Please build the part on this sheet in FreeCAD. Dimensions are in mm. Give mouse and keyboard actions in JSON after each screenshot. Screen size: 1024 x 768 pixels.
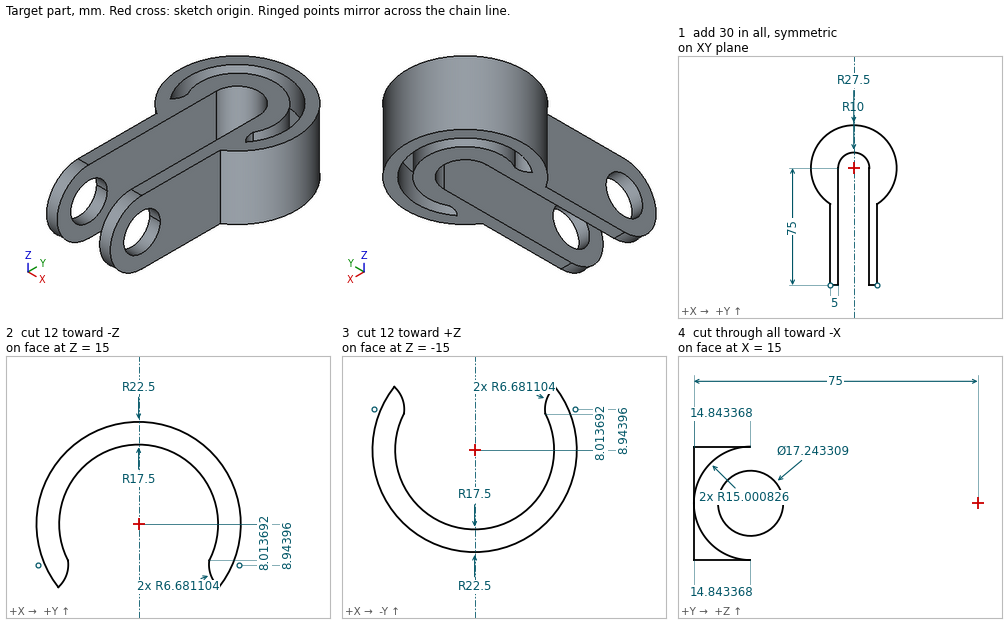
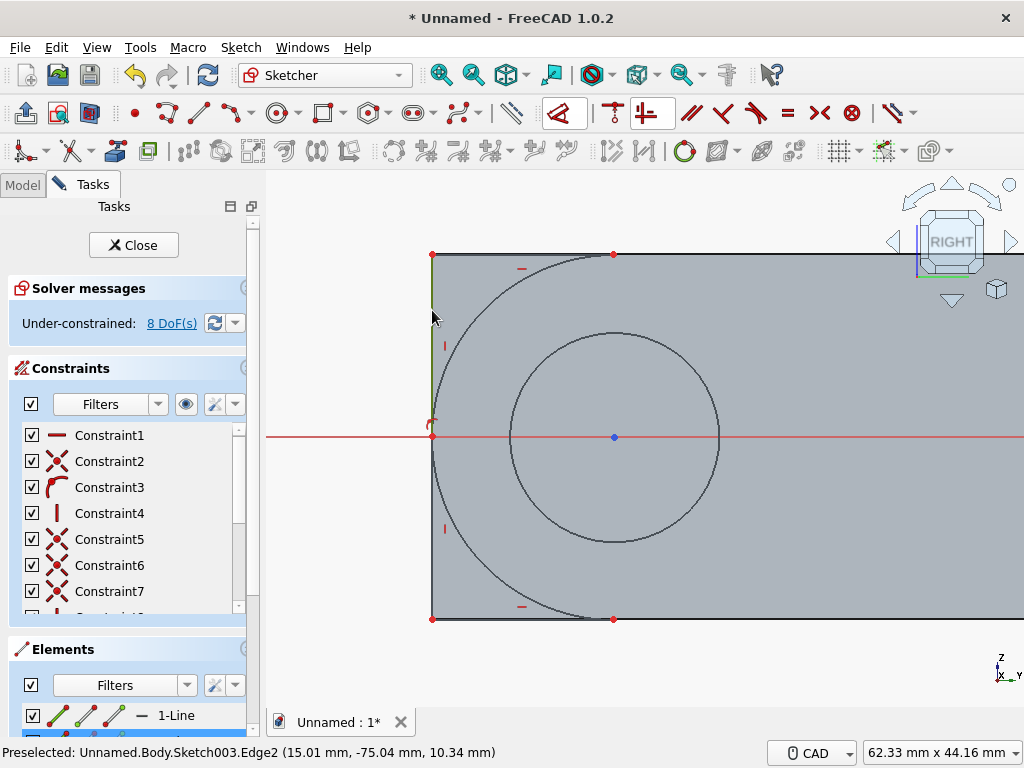
{"action": "left_click", "coordinate": [531, 275]}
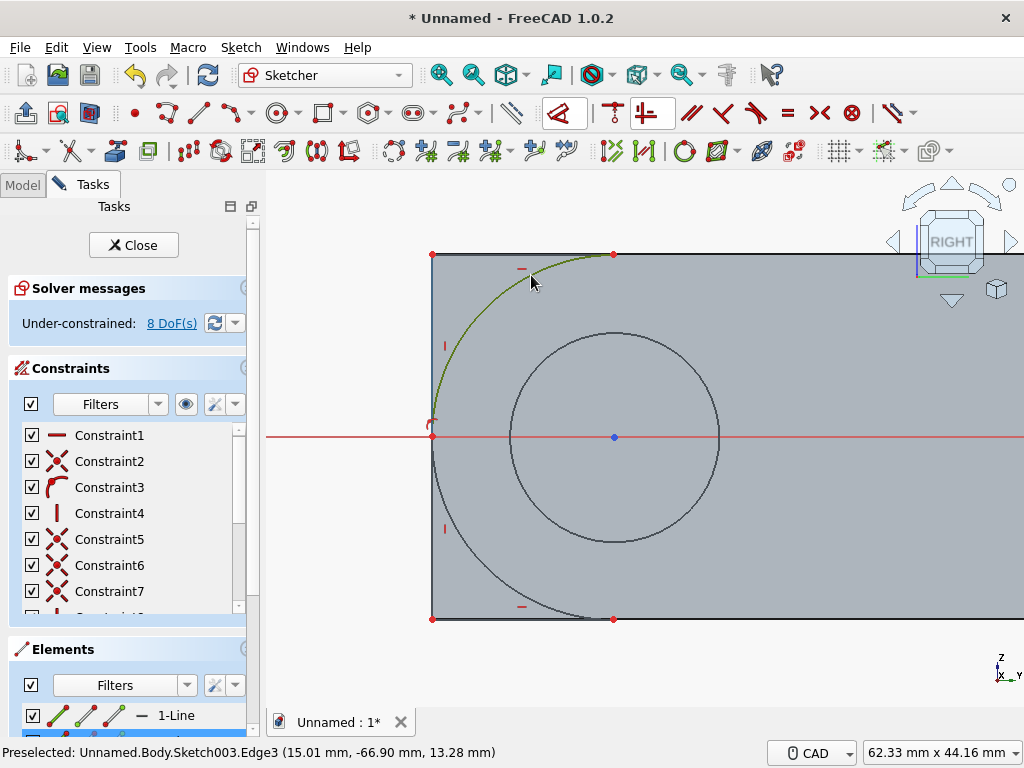
{"action": "left_click", "coordinate": [756, 114]}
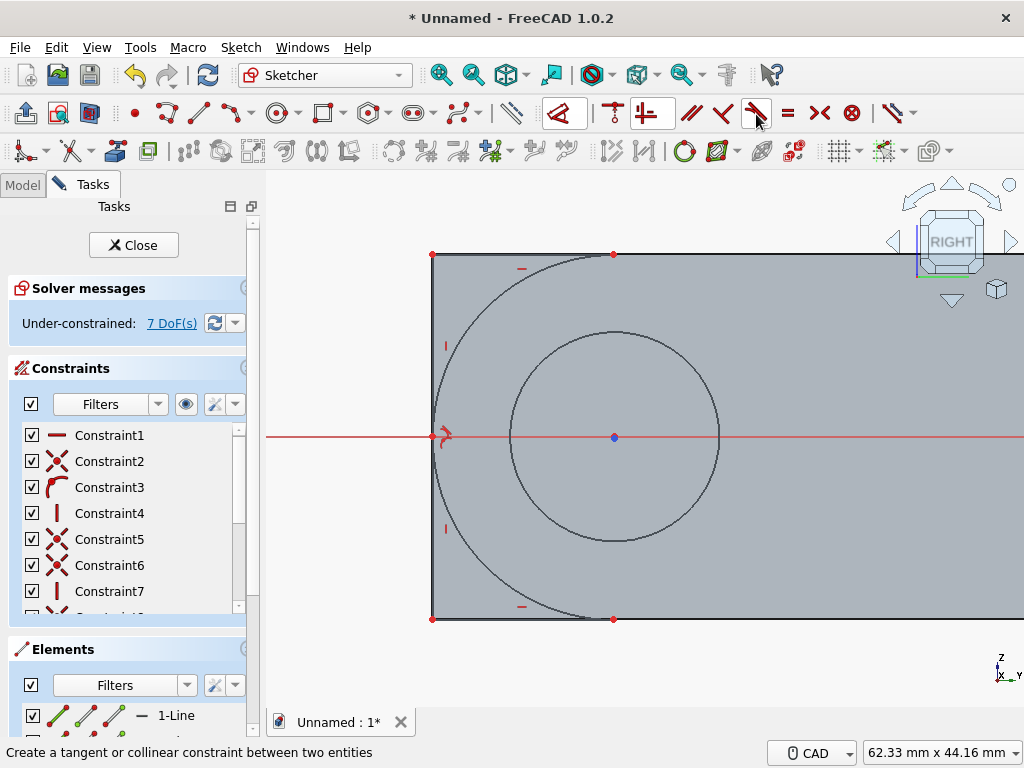
{"action": "left_click", "coordinate": [433, 310]}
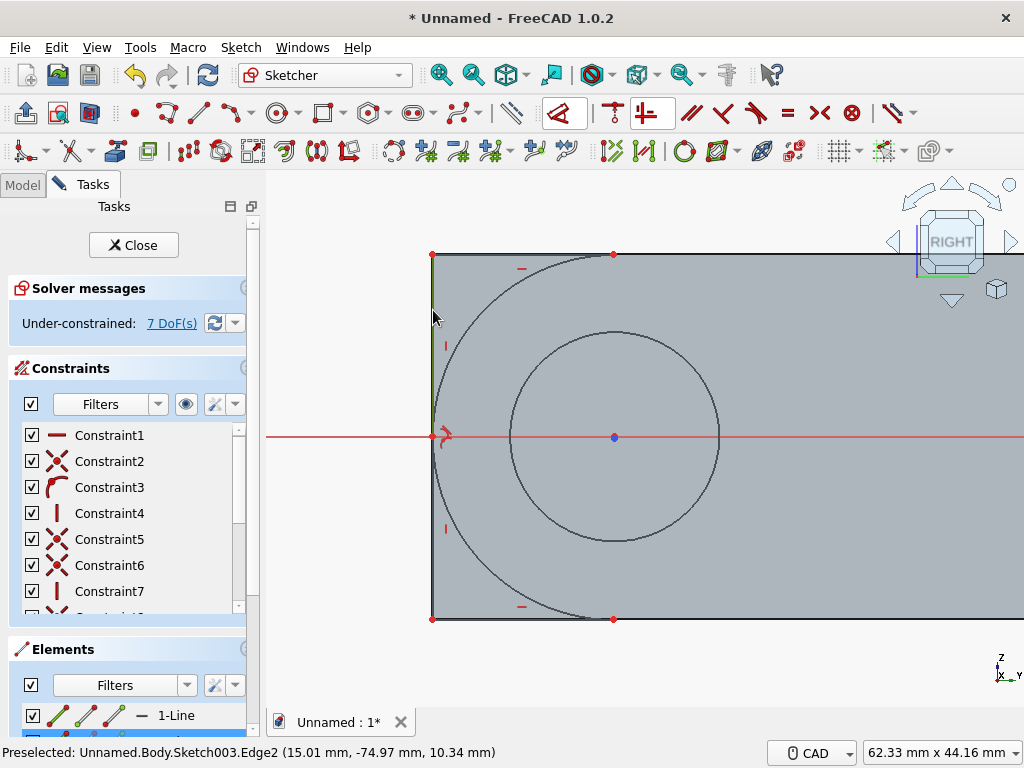
{"action": "left_click", "coordinate": [452, 519]}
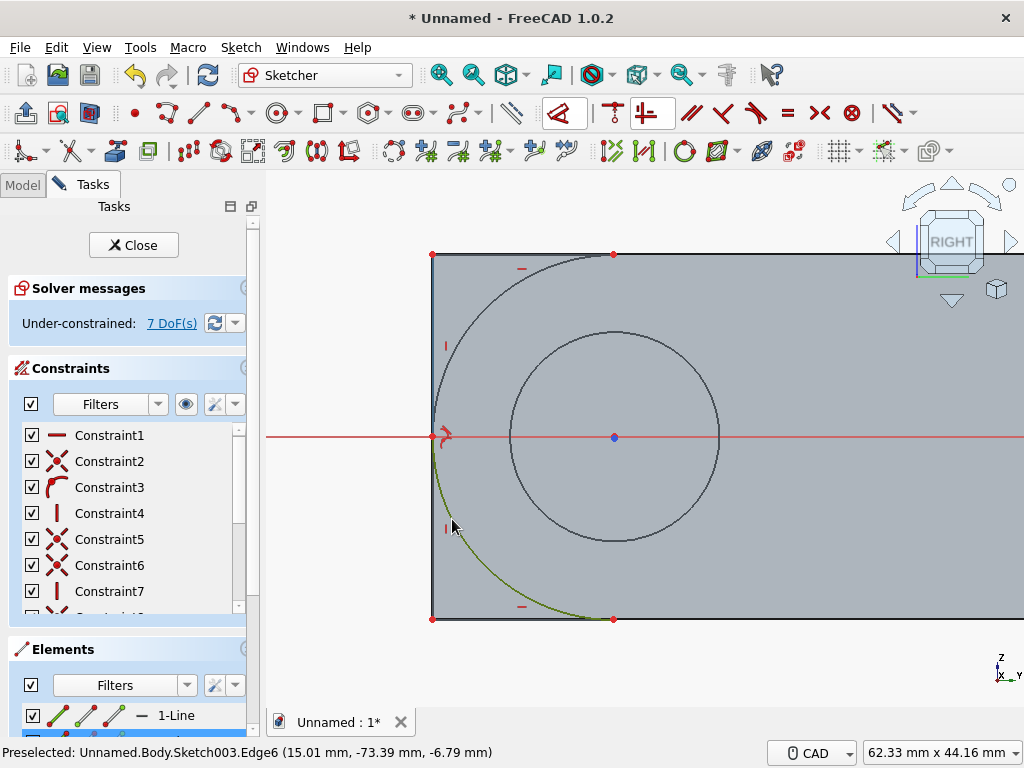
{"action": "left_click", "coordinate": [756, 114]}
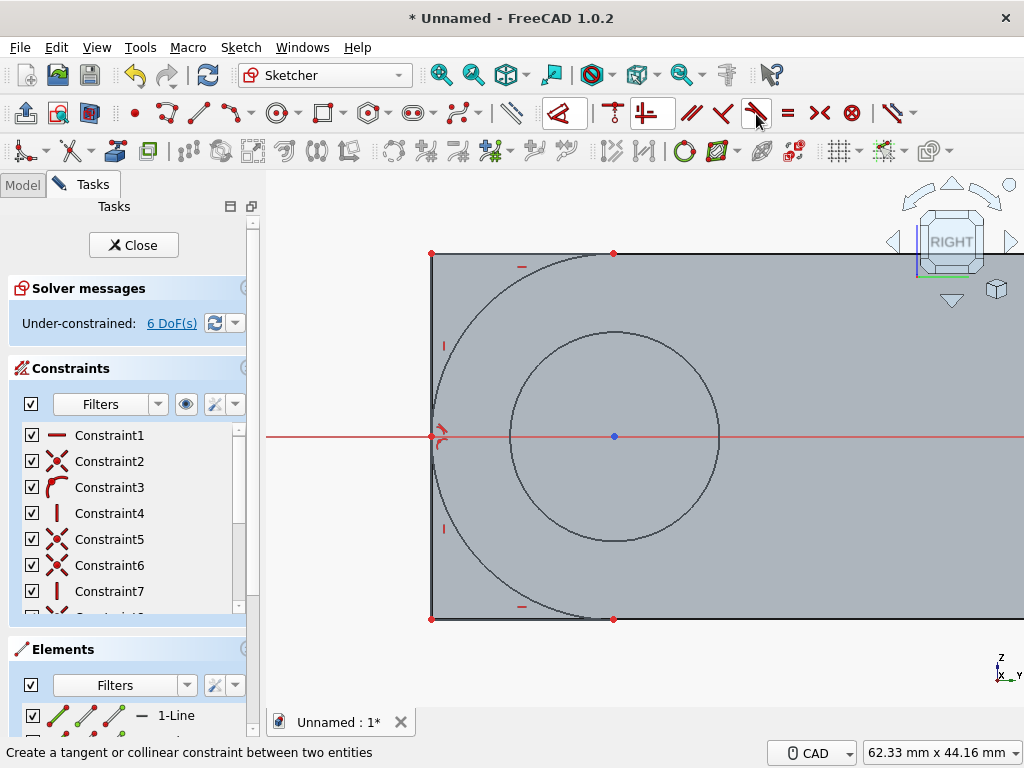
{"action": "left_click", "coordinate": [530, 274]}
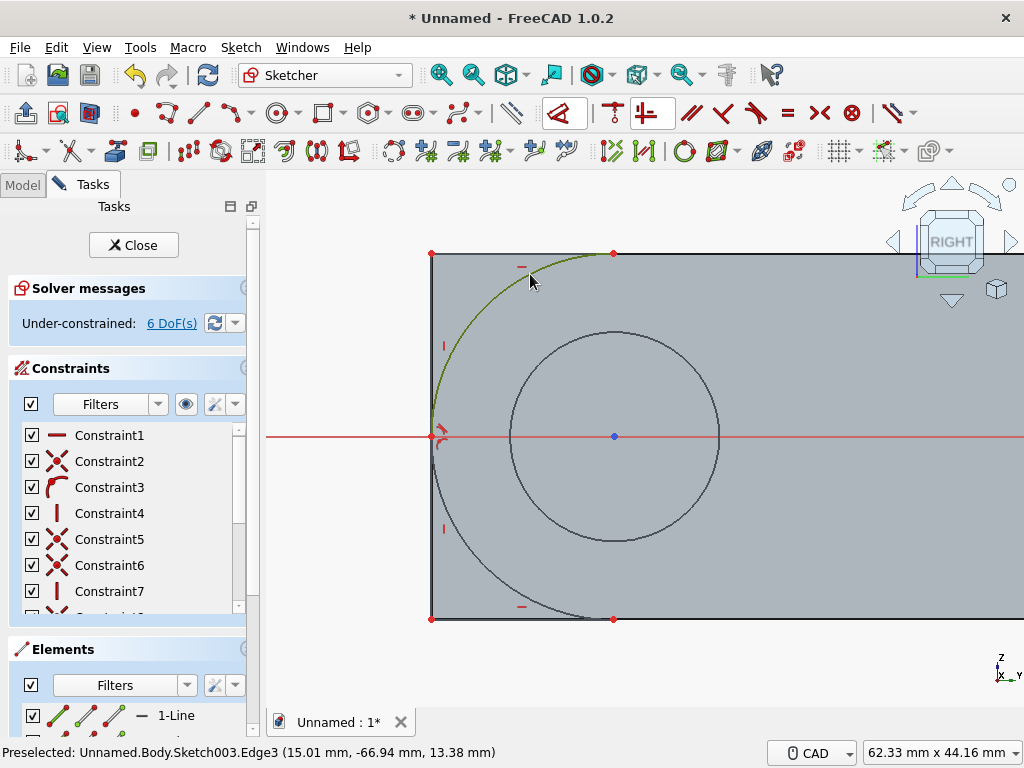
{"action": "left_click", "coordinate": [451, 520]}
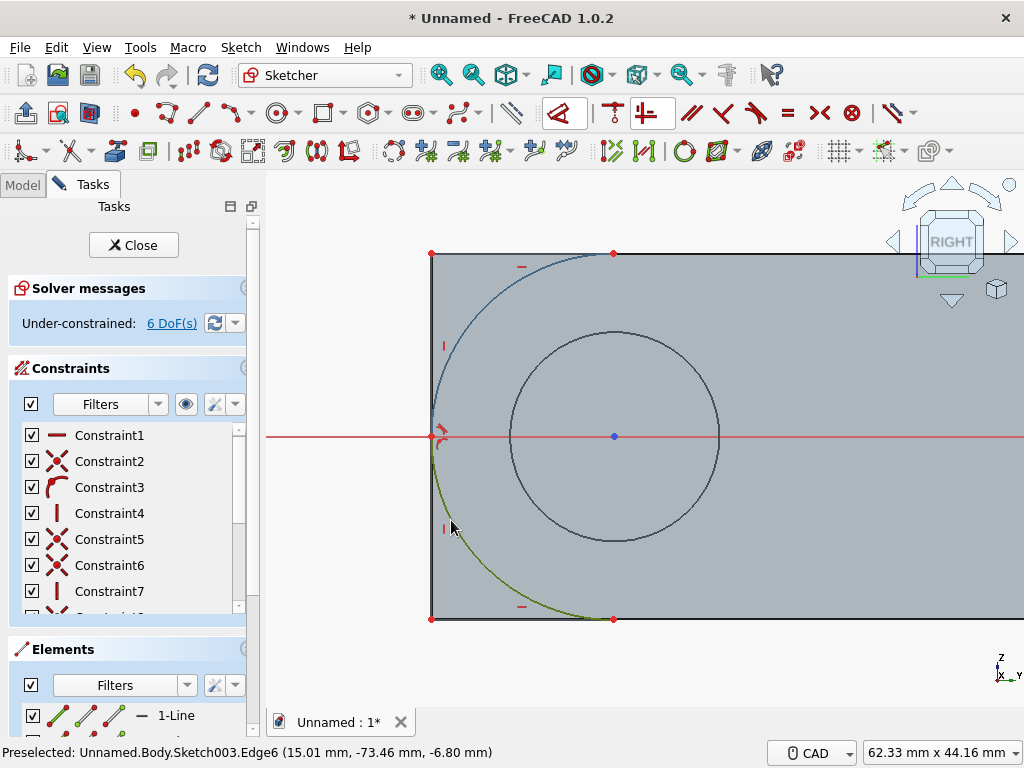
{"action": "key", "text": "e"}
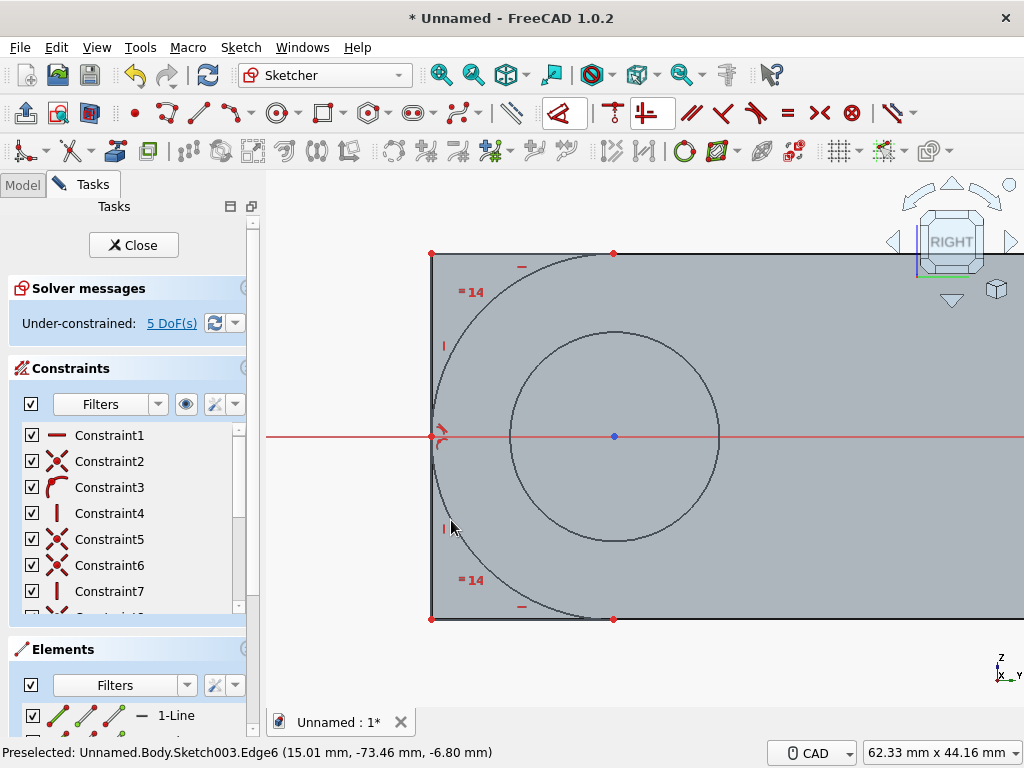
{"action": "left_click", "coordinate": [530, 274]}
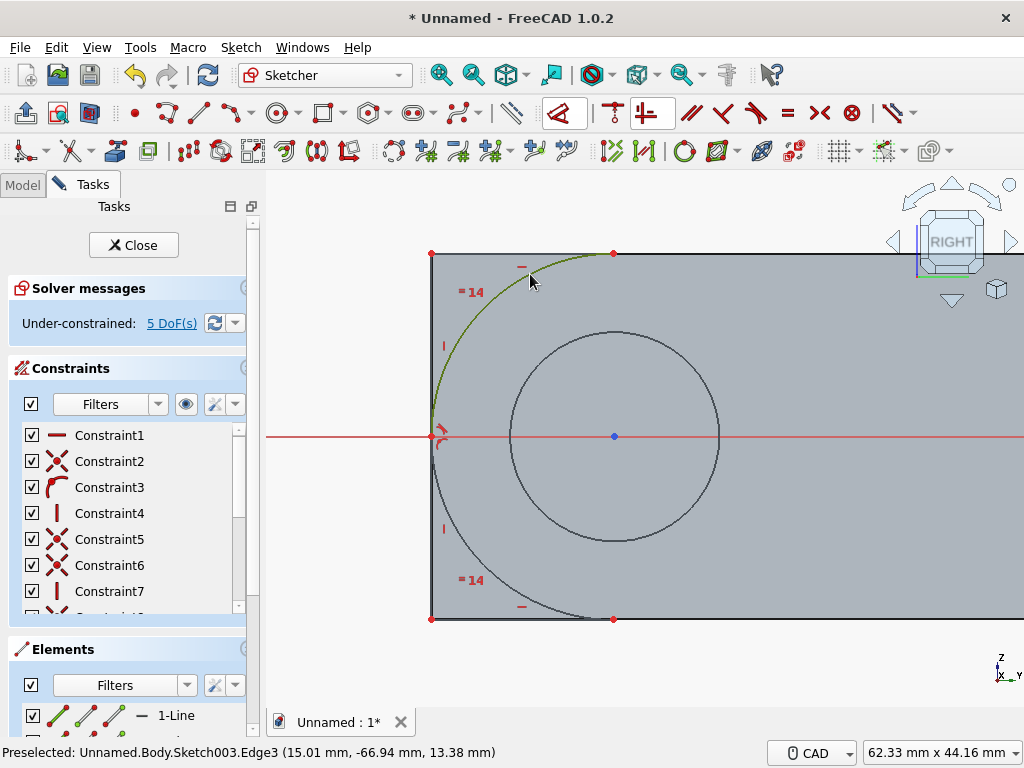
{"action": "left_click", "coordinate": [582, 114]}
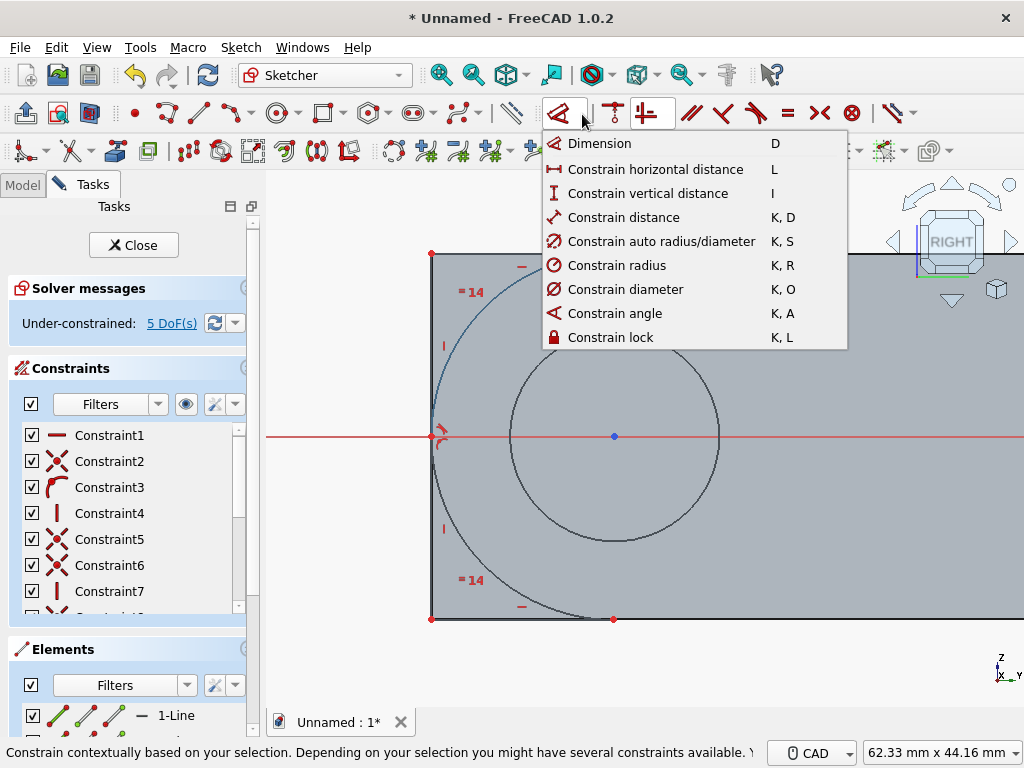
{"action": "left_click", "coordinate": [695, 265]}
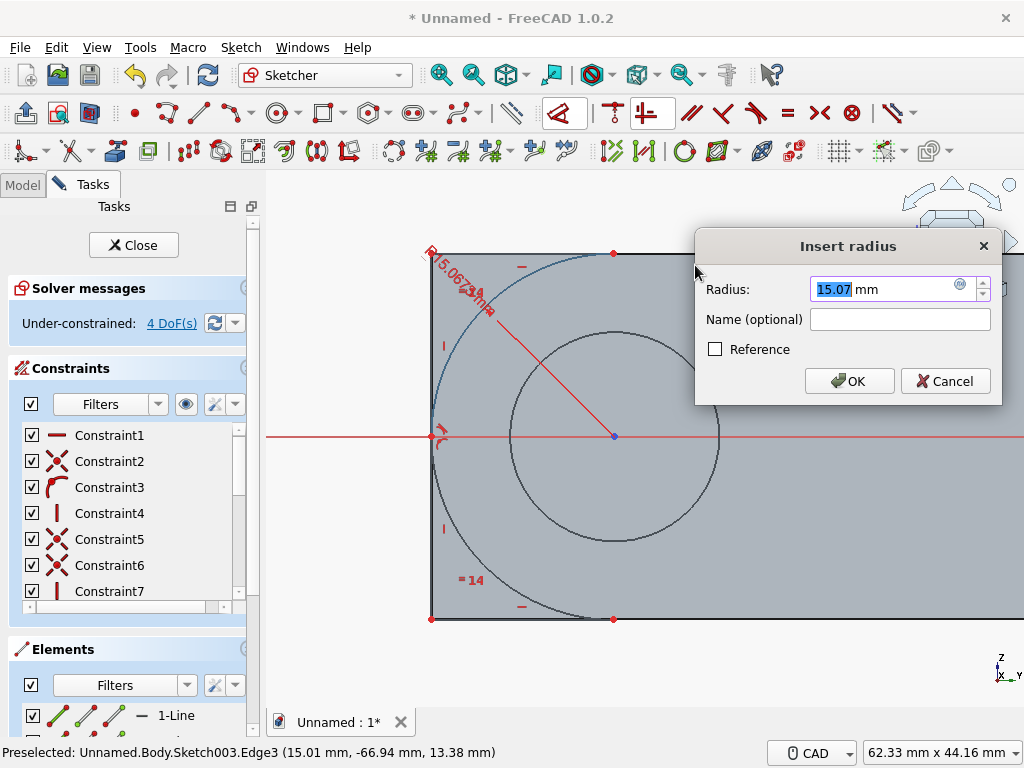
{"action": "type", "text": "15.000826"}
{"action": "key", "text": "Return"}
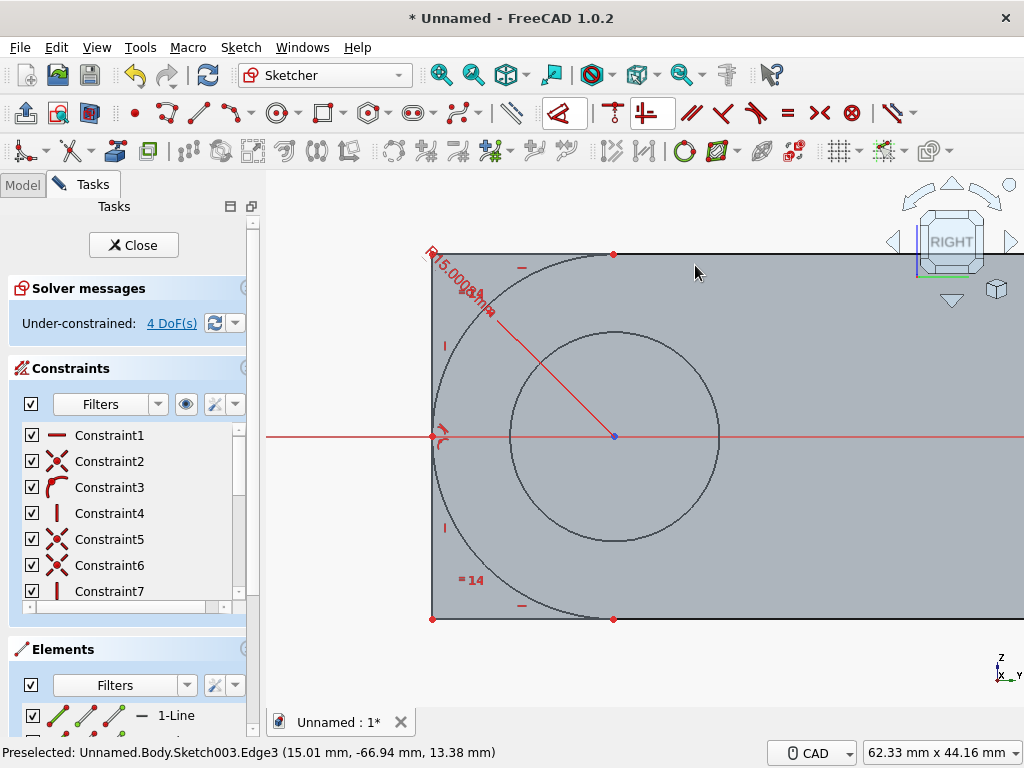
{"action": "left_click", "coordinate": [688, 363]}